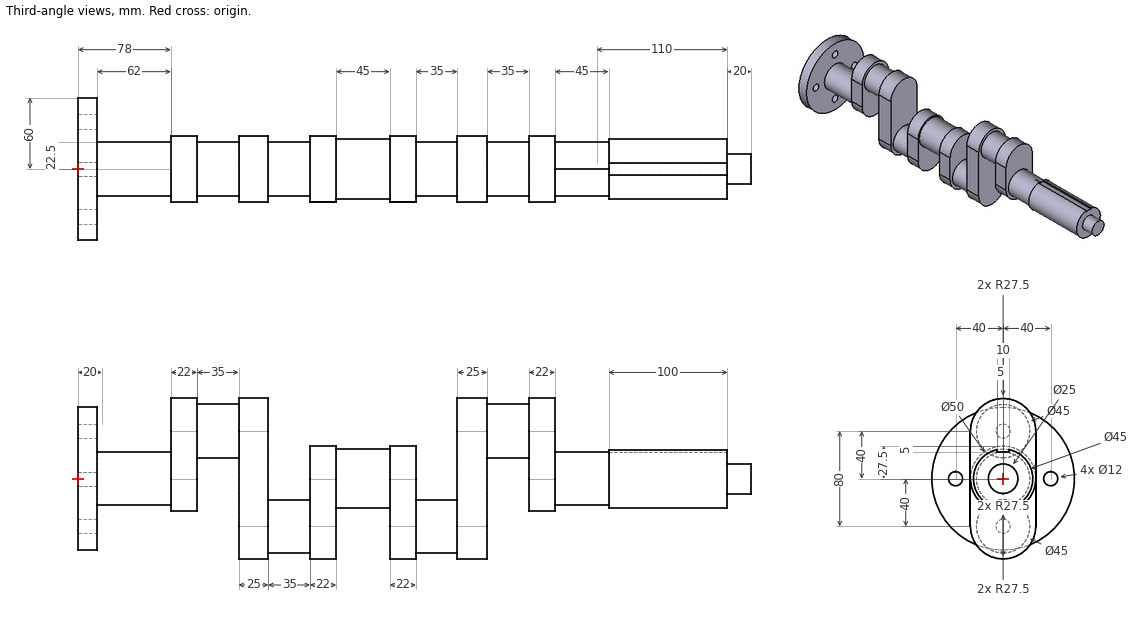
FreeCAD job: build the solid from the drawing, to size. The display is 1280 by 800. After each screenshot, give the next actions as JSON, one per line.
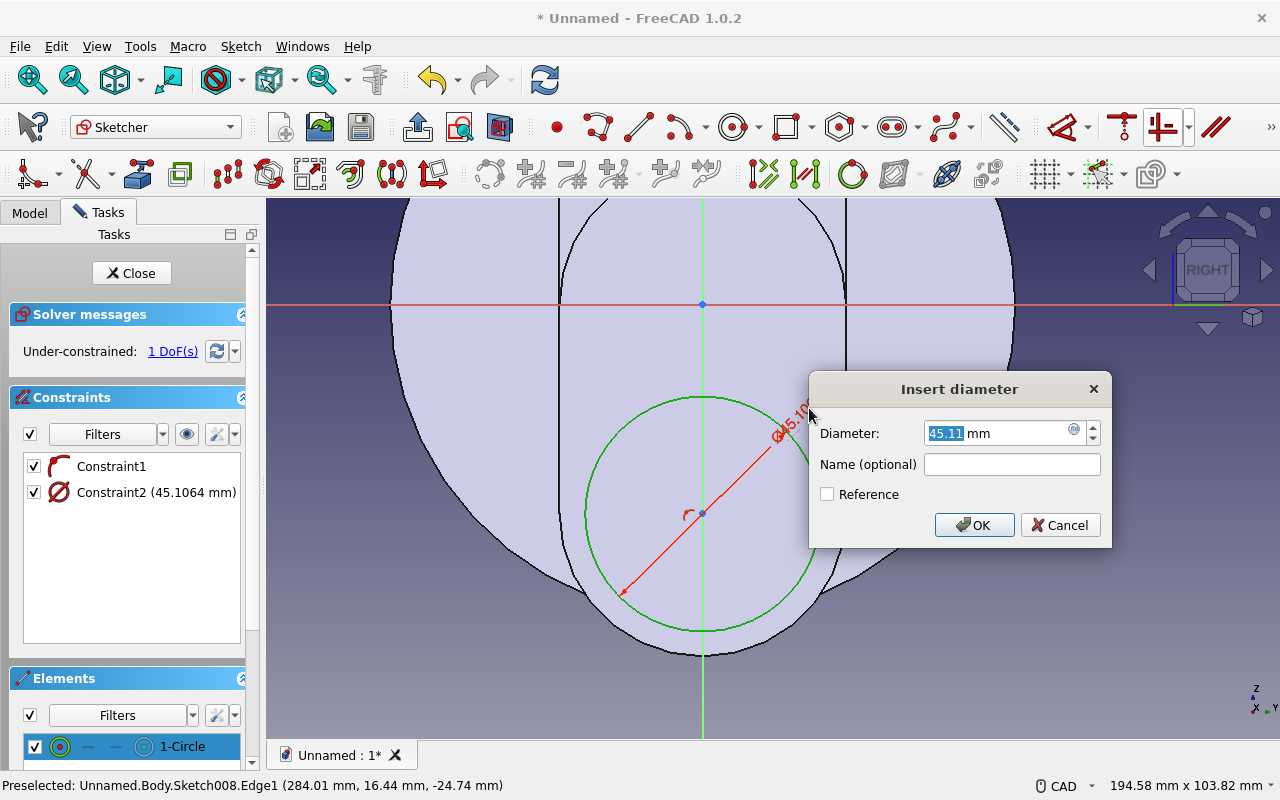
{"action": "type", "text": "45"}
{"action": "key", "text": "Return"}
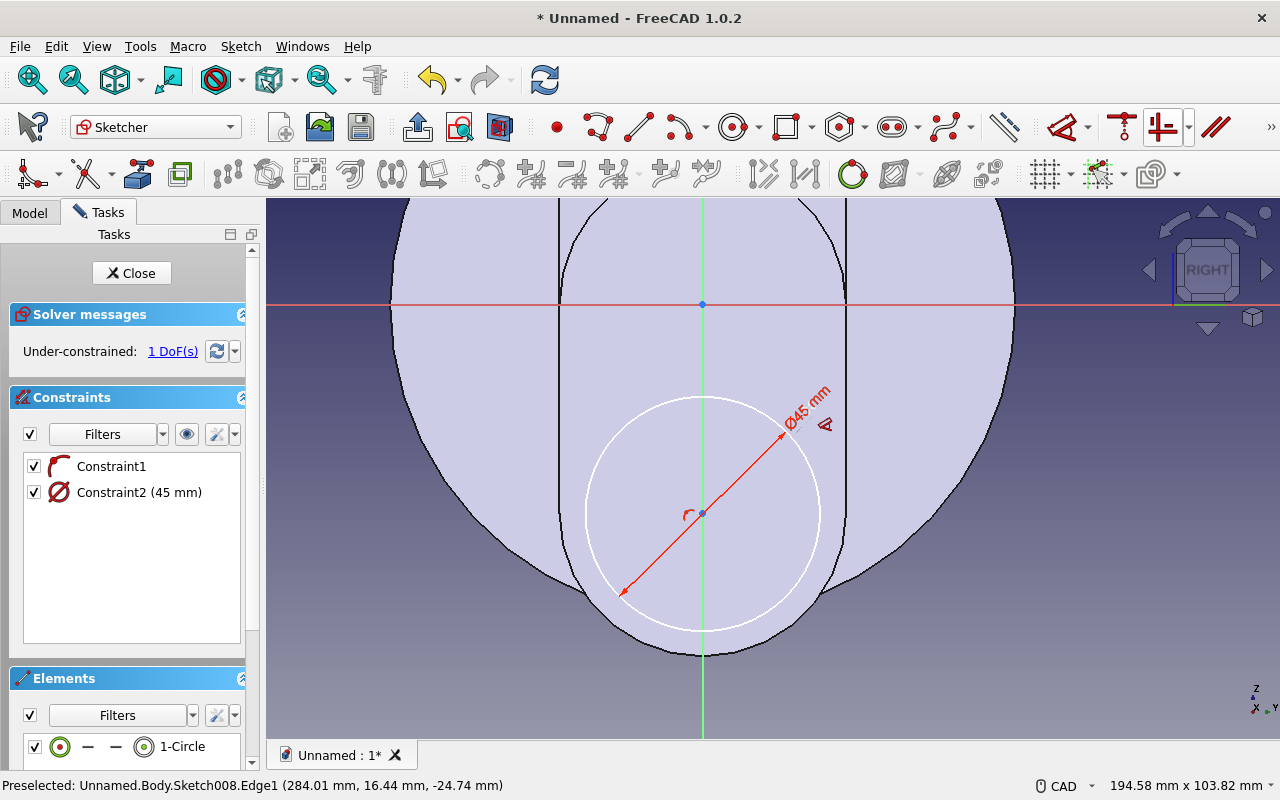
{"action": "left_click", "coordinate": [703, 514]}
{"action": "left_click", "coordinate": [737, 361]}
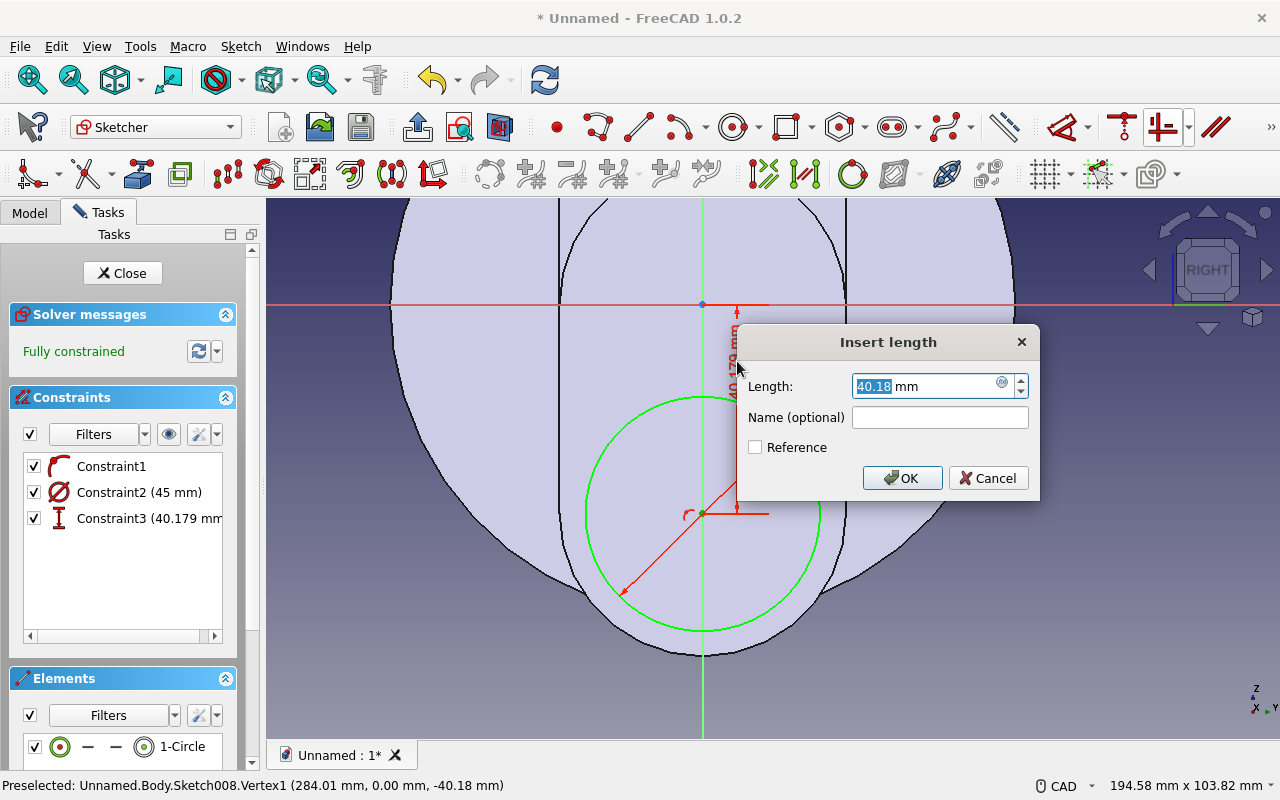
{"action": "type", "text": "40"}
{"action": "key", "text": "Return"}
{"action": "key", "text": "Escape"}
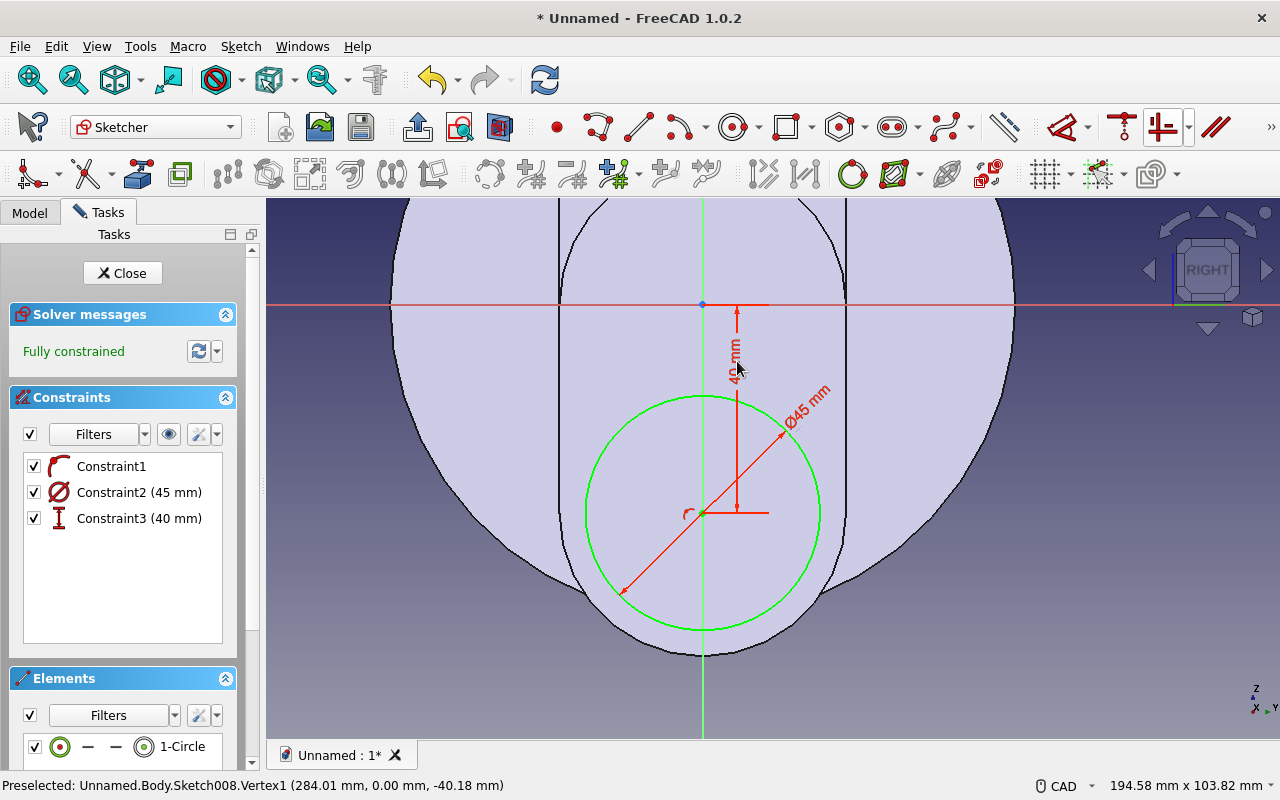
{"action": "left_click", "coordinate": [123, 273]}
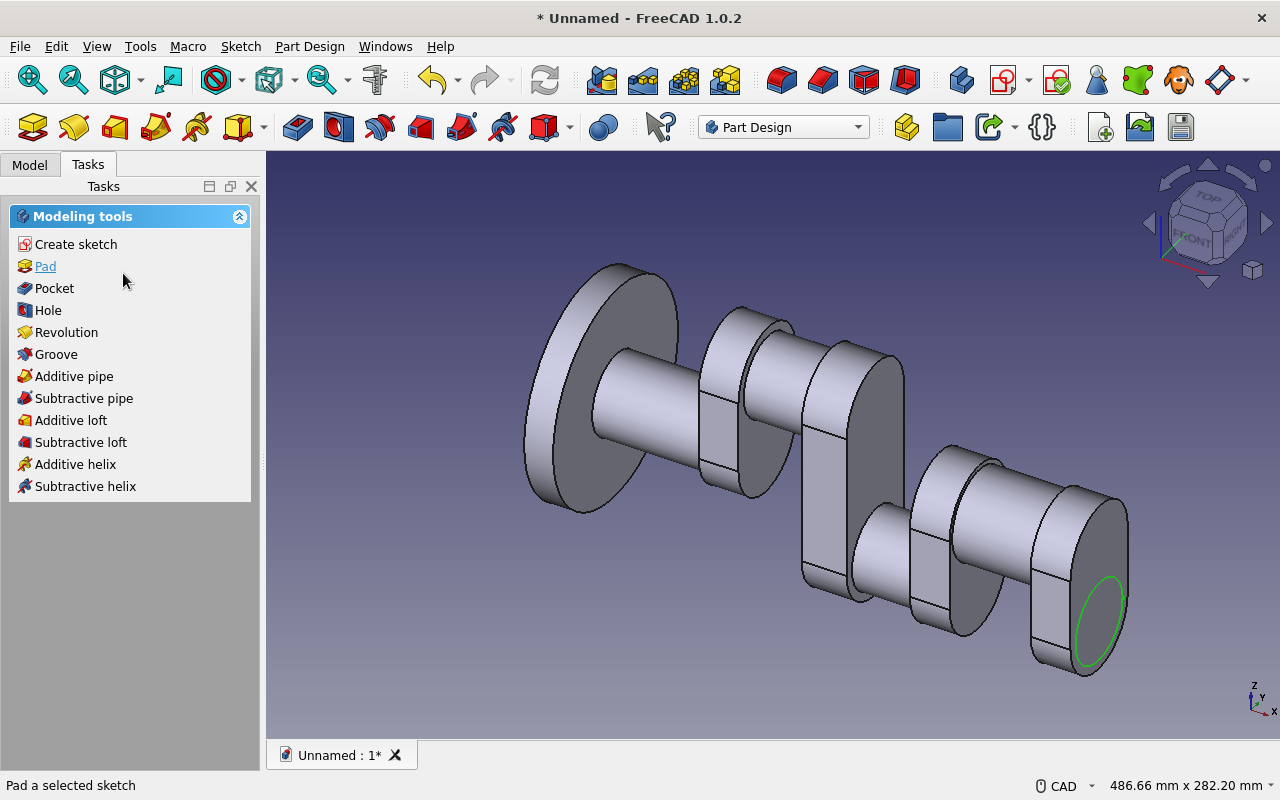
{"action": "left_click", "coordinate": [33, 128]}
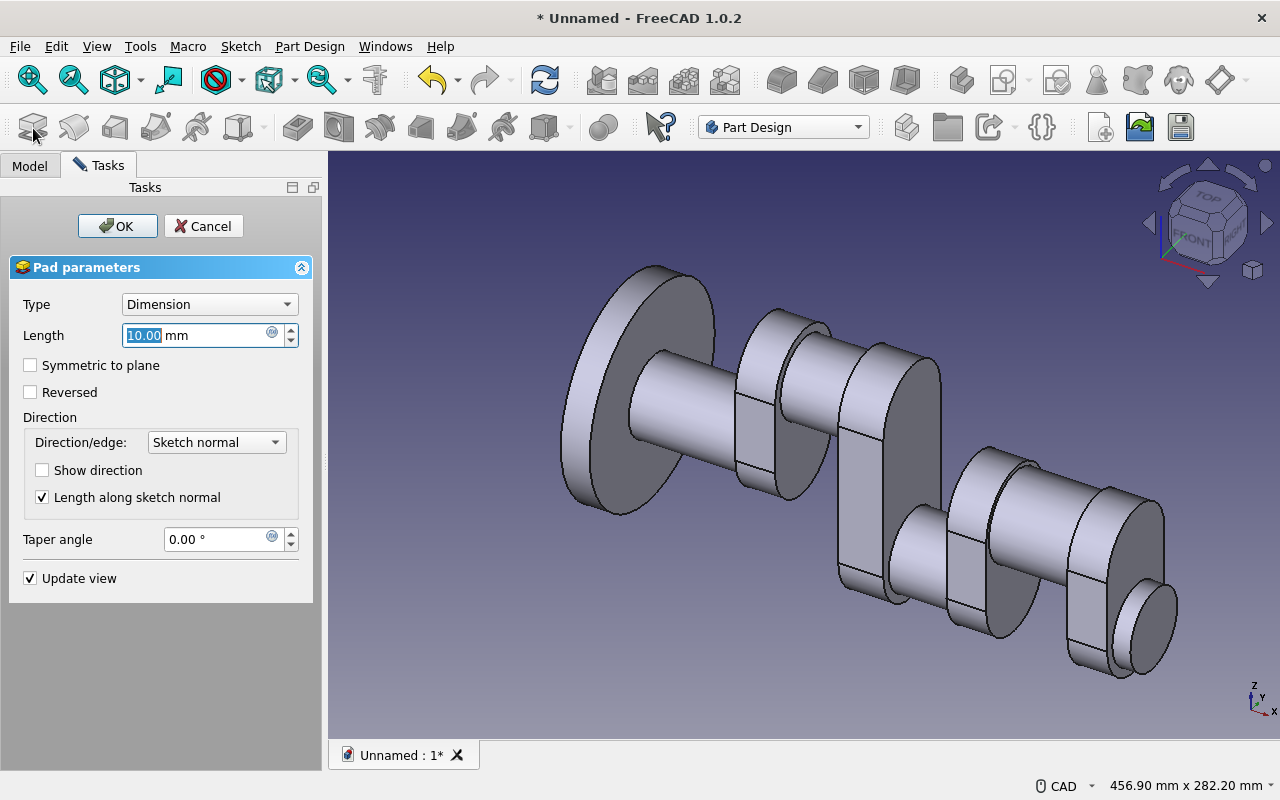
{"action": "type", "text": "35"}
{"action": "key", "text": "Tab"}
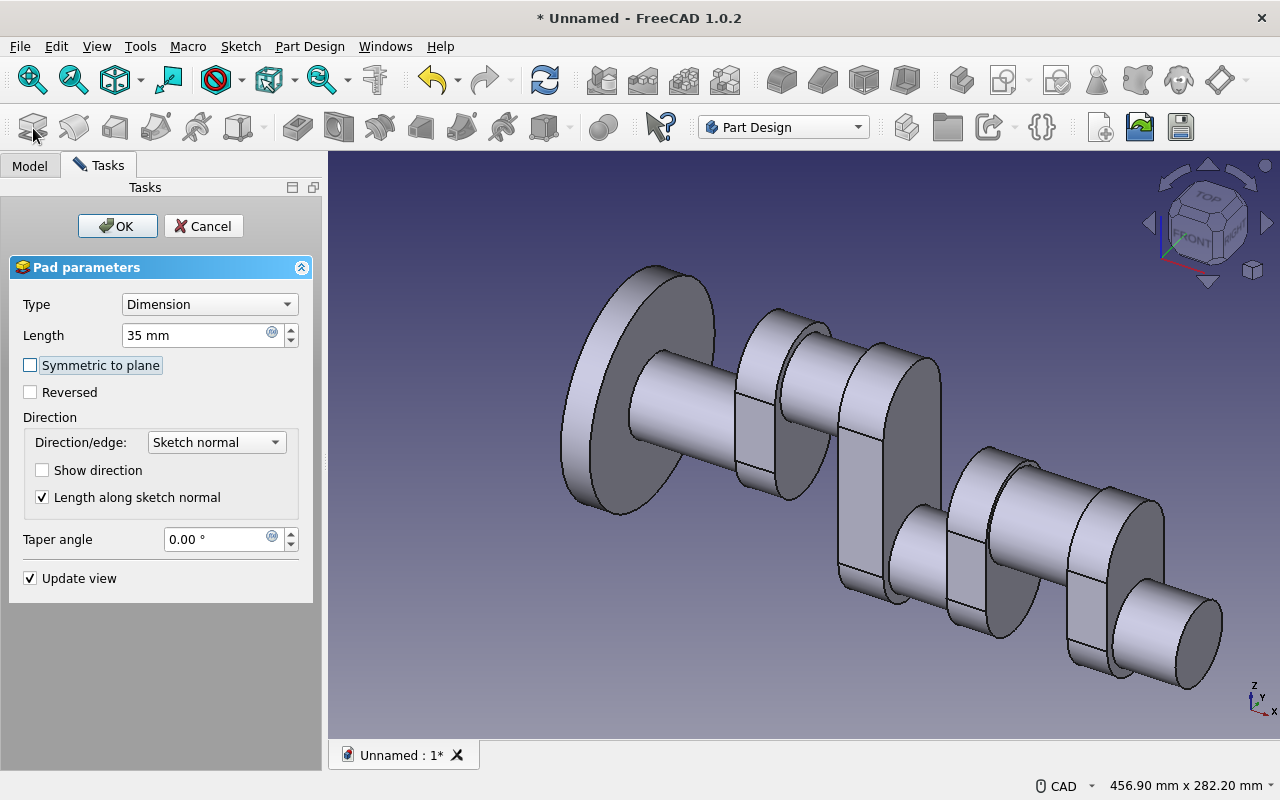
{"action": "left_click", "coordinate": [118, 226]}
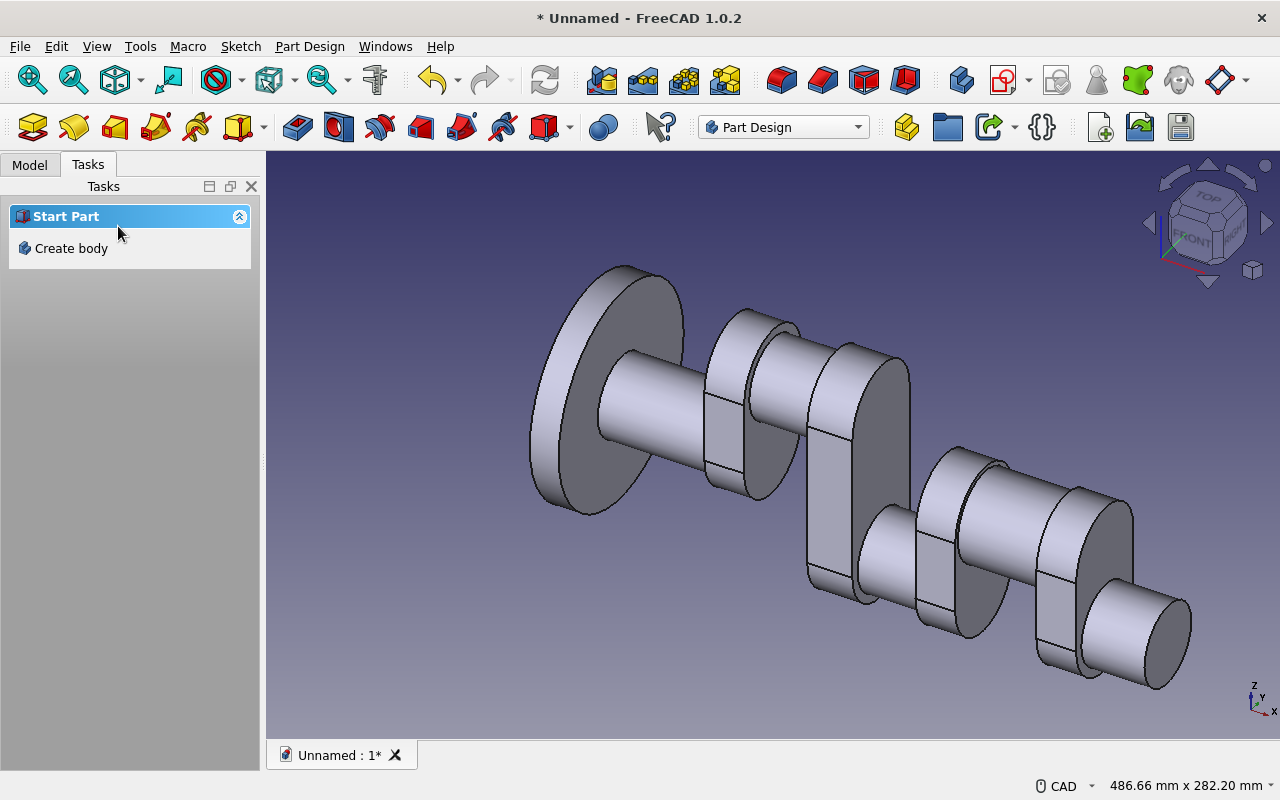
{"action": "key", "text": "v f"}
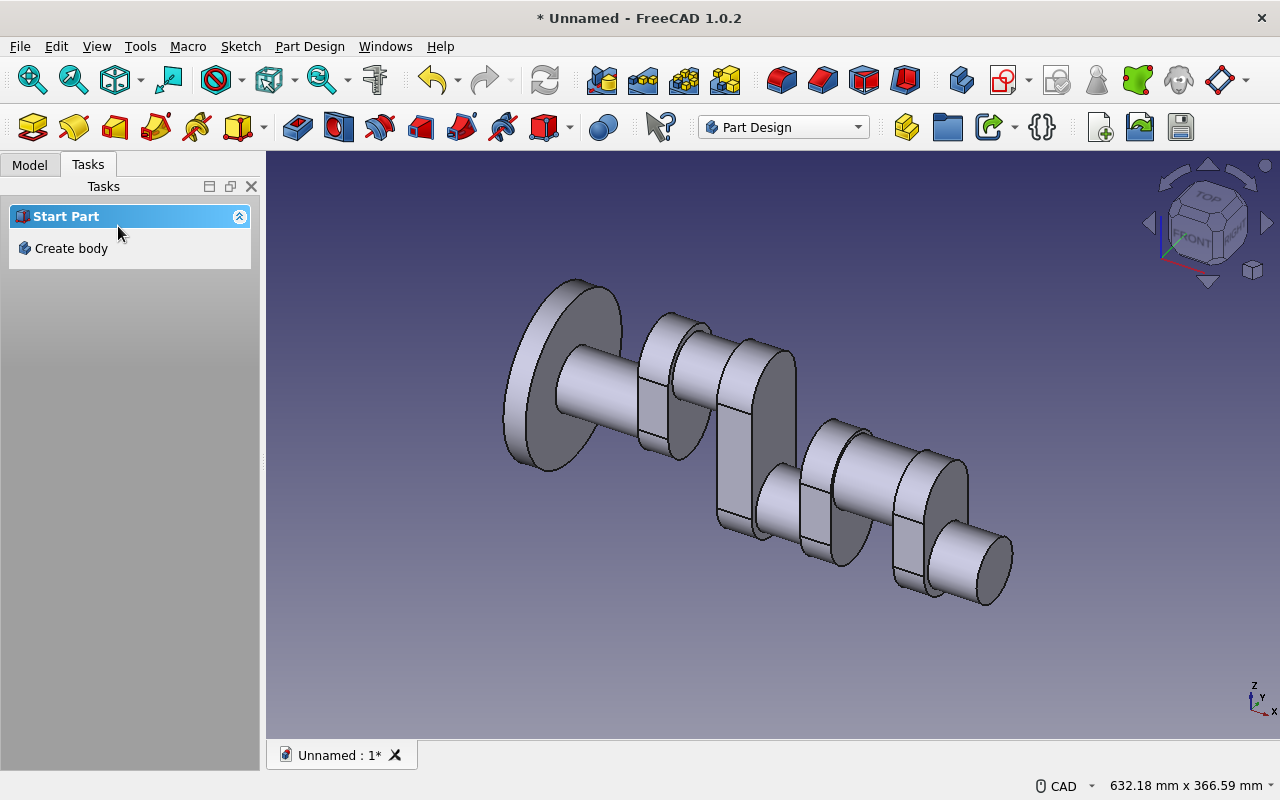
{"action": "left_click", "coordinate": [995, 570]}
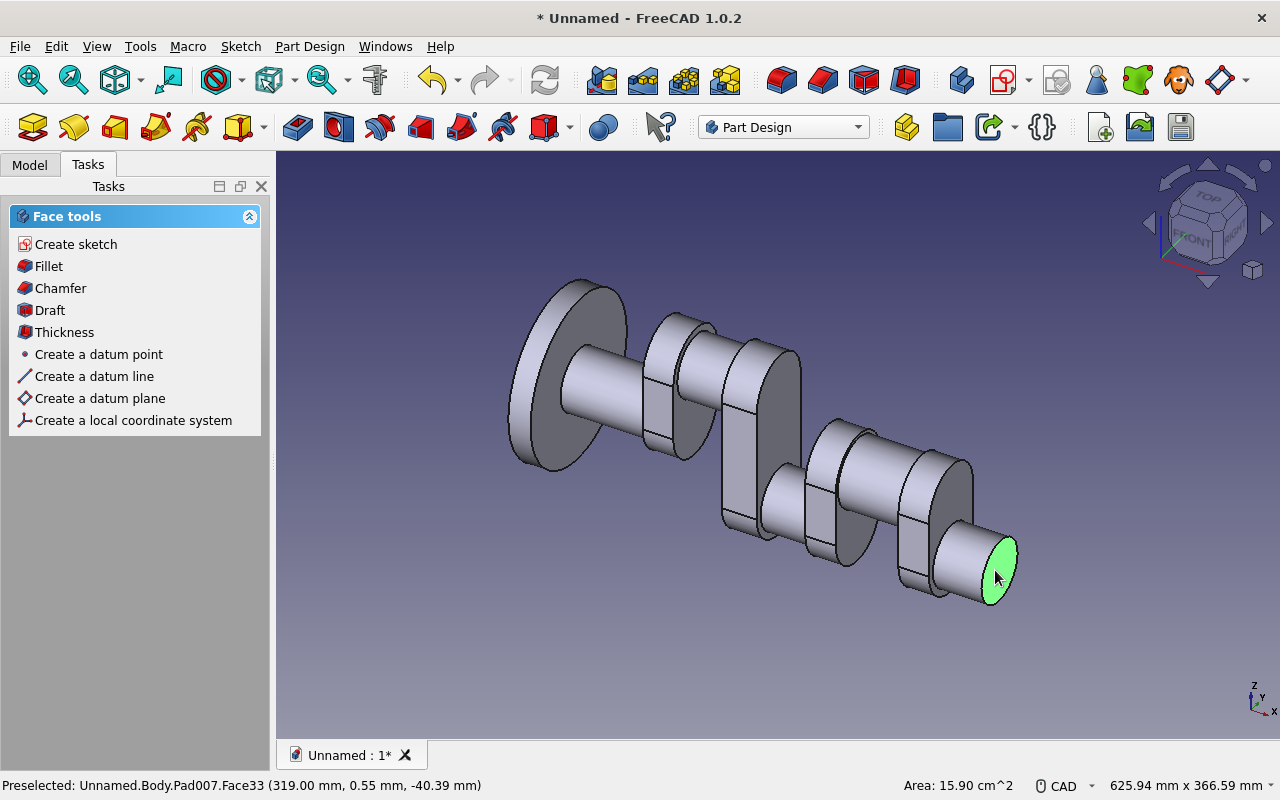
{"action": "left_click", "coordinate": [1002, 80]}